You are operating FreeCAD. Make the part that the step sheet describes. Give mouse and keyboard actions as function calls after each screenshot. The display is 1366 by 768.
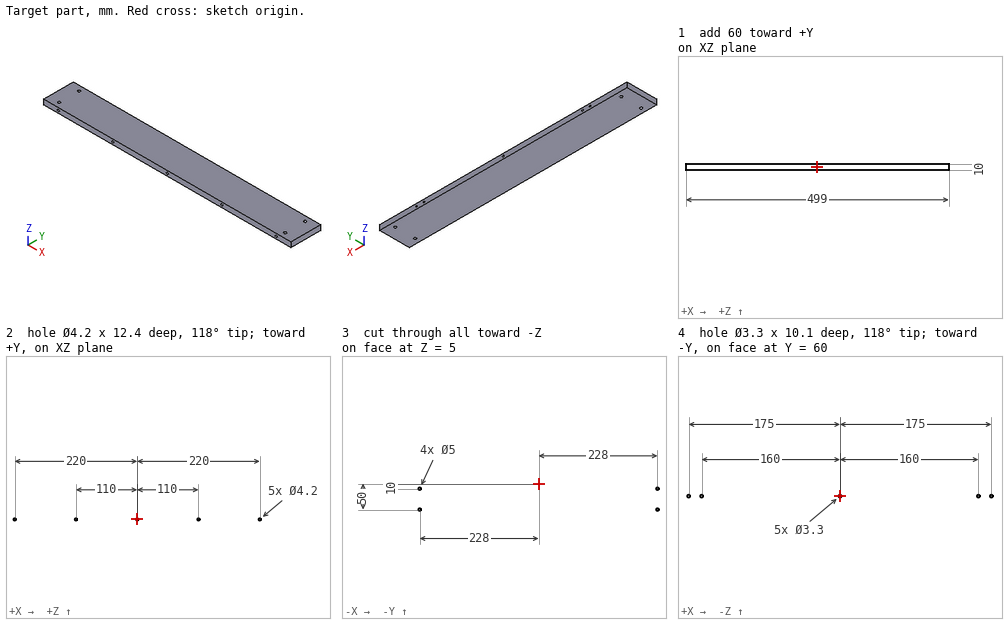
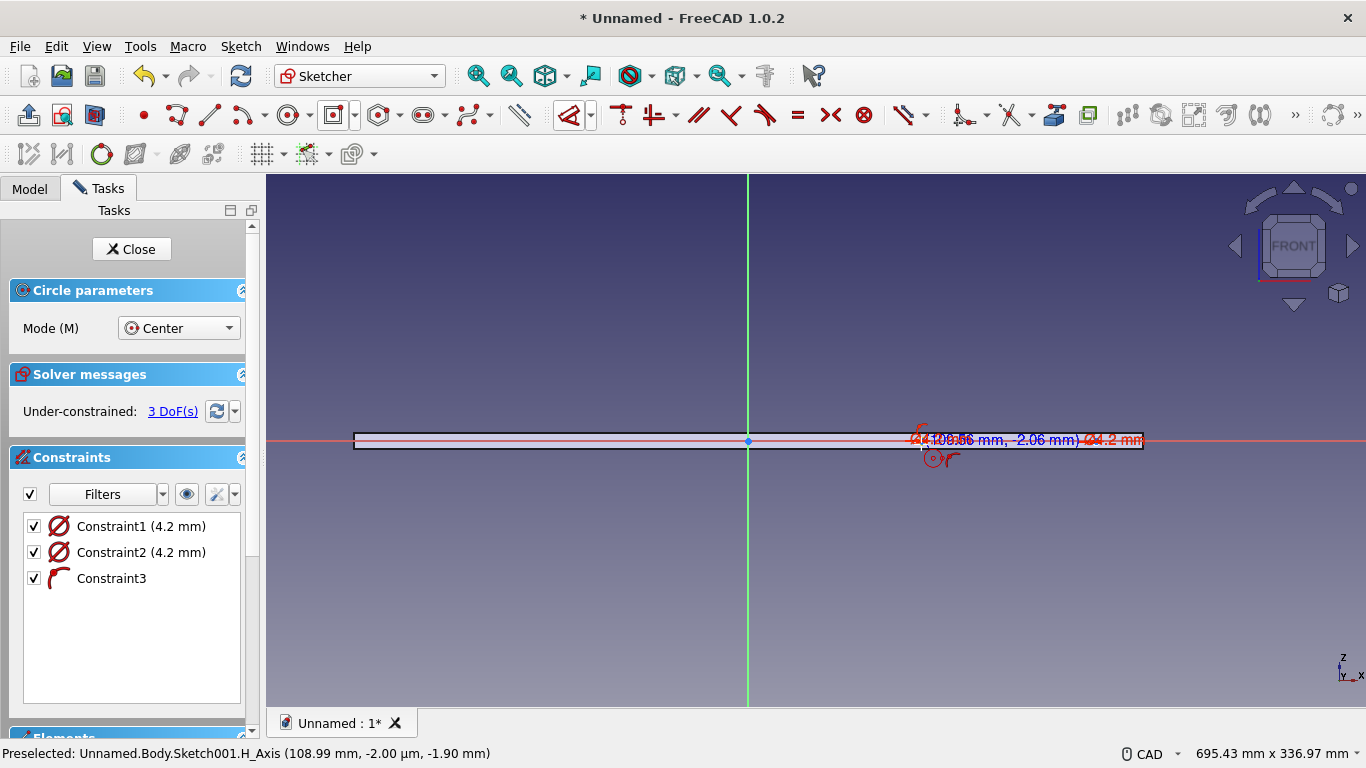
scroll(748, 441, up, 10)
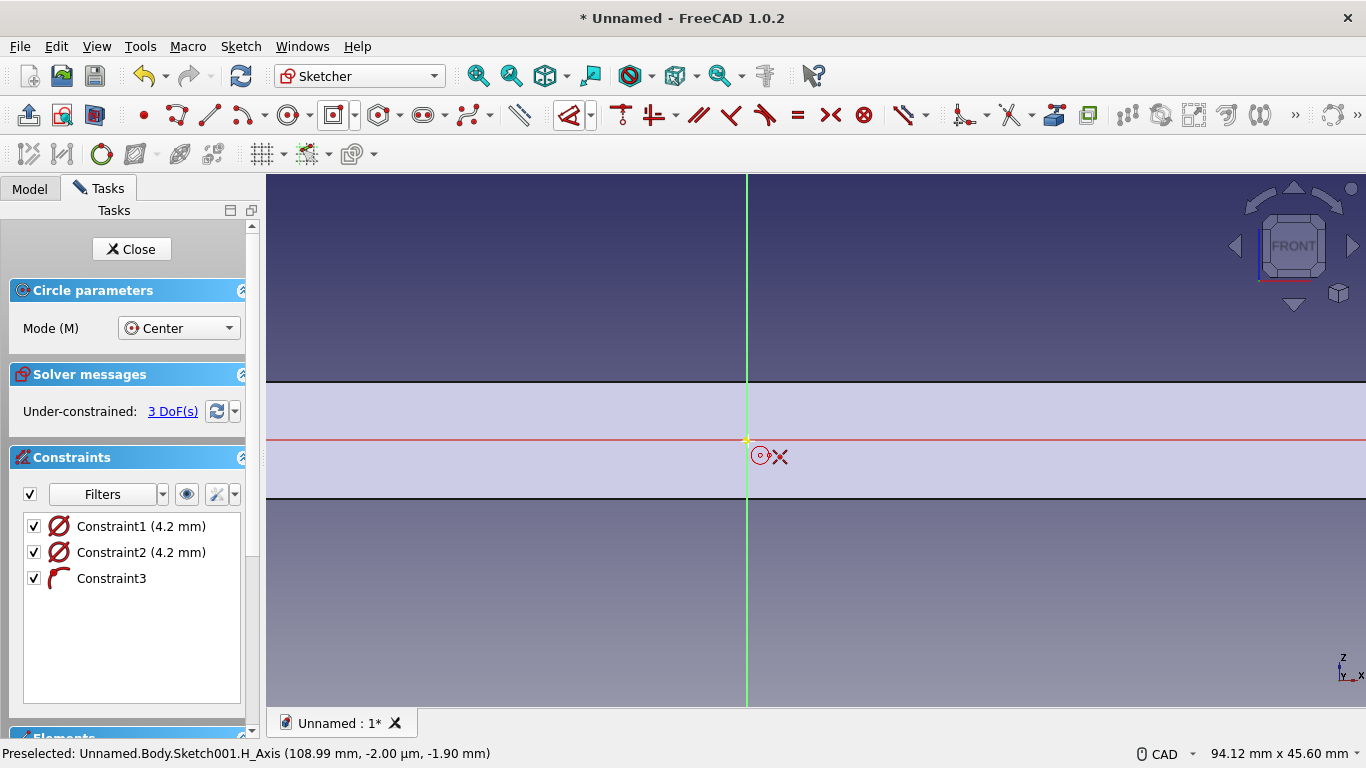
scroll(748, 441, down, 10)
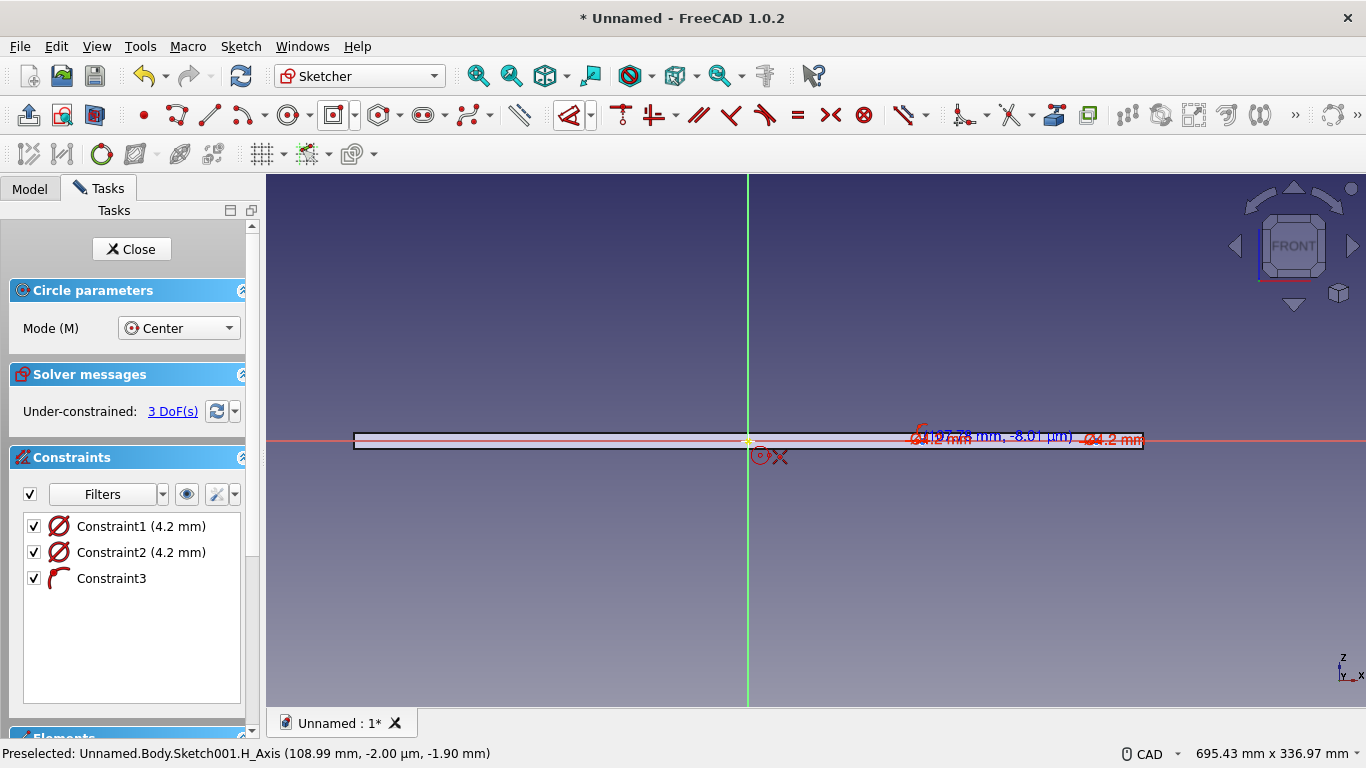
click(748, 441)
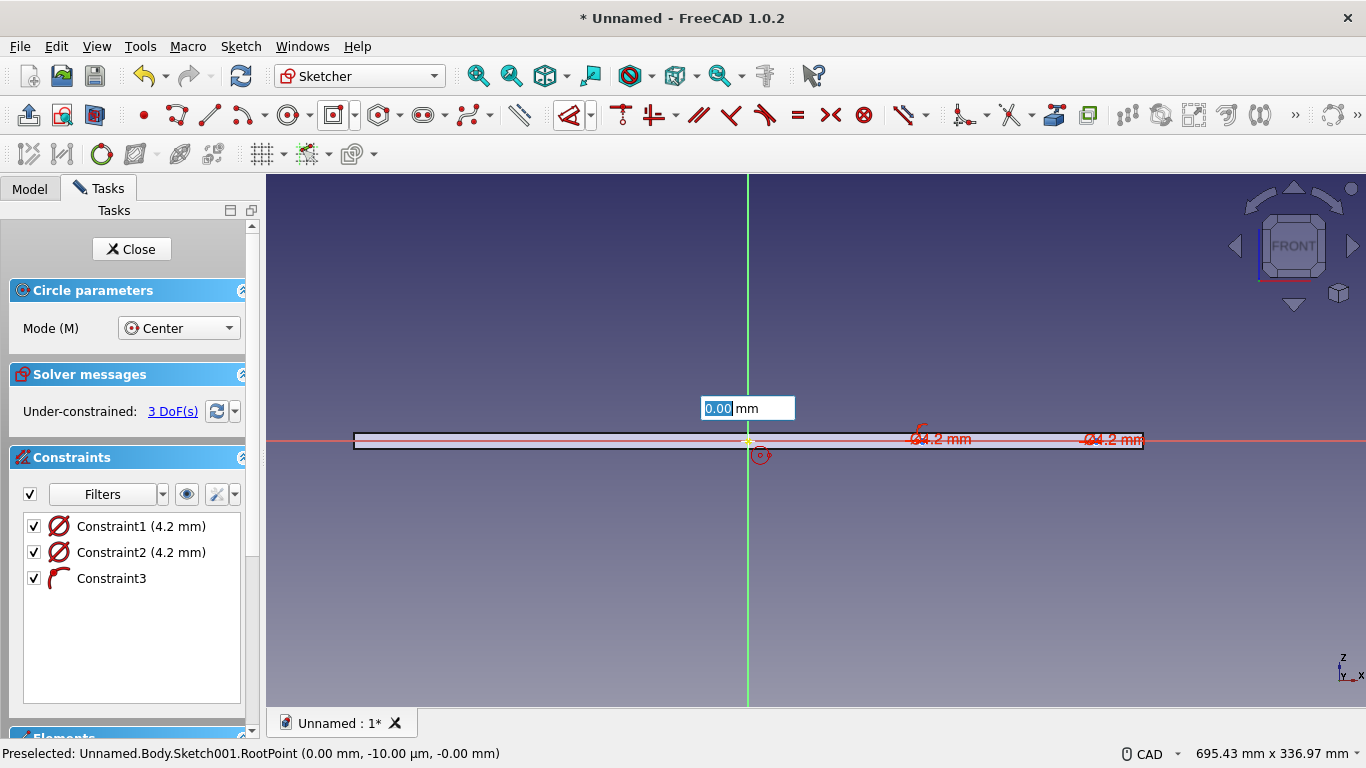
scroll(751, 439, up, 10)
move(745, 436)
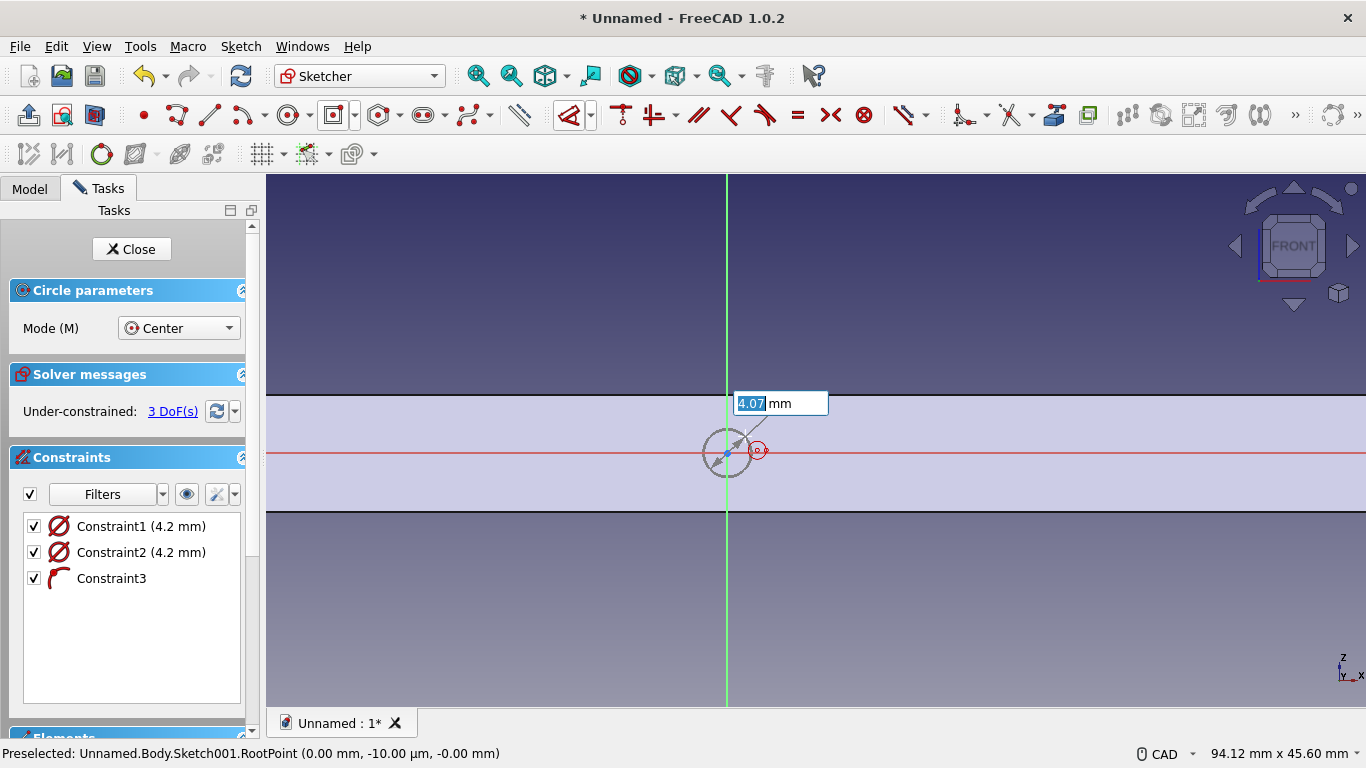
text(4.2)
key(Return)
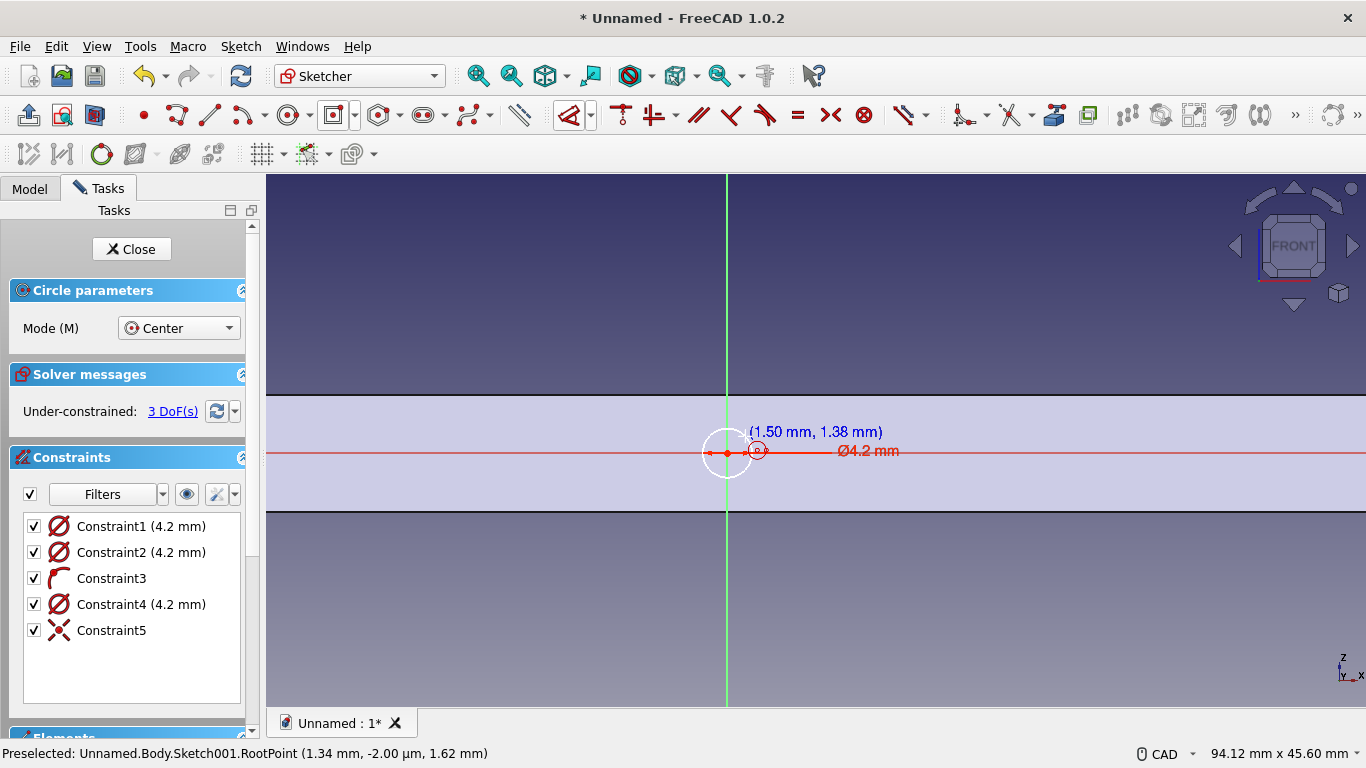
scroll(751, 439, down, 10)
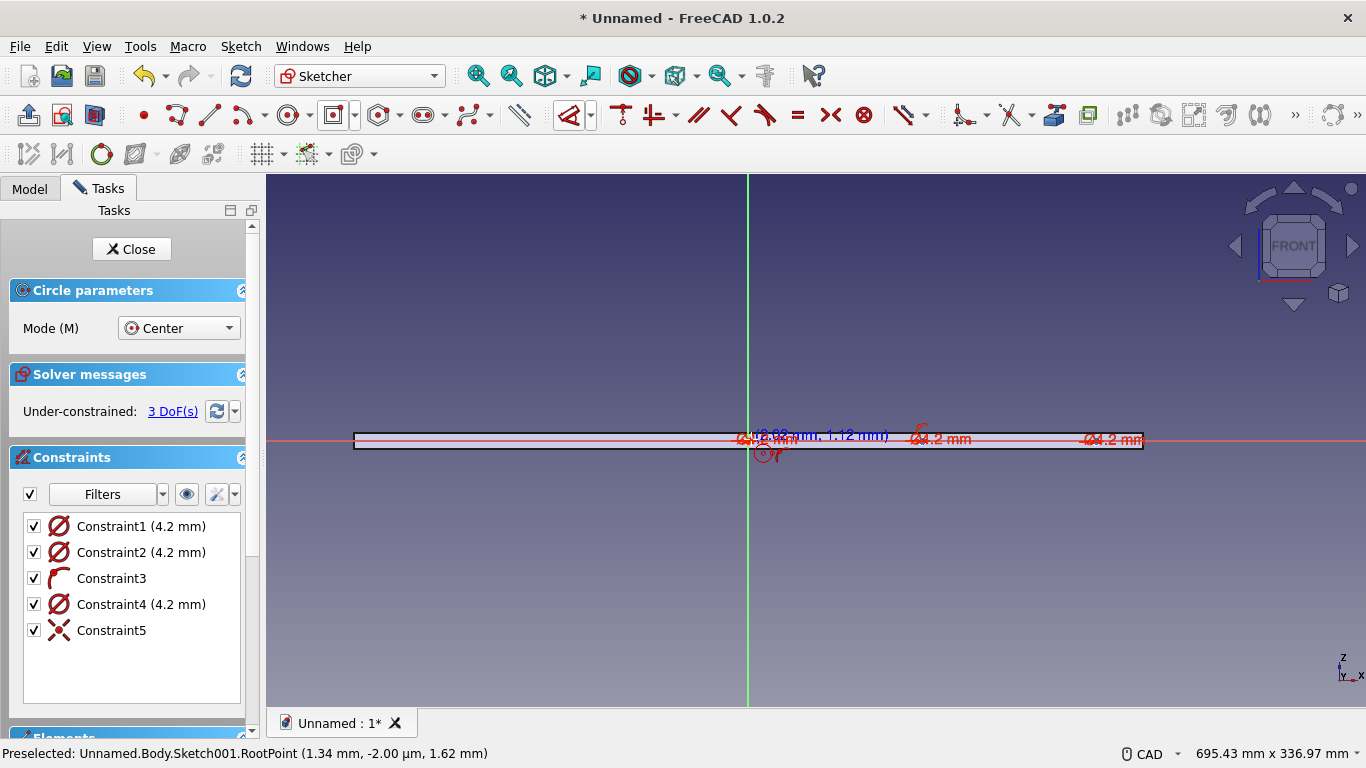
scroll(574, 441, up, 10)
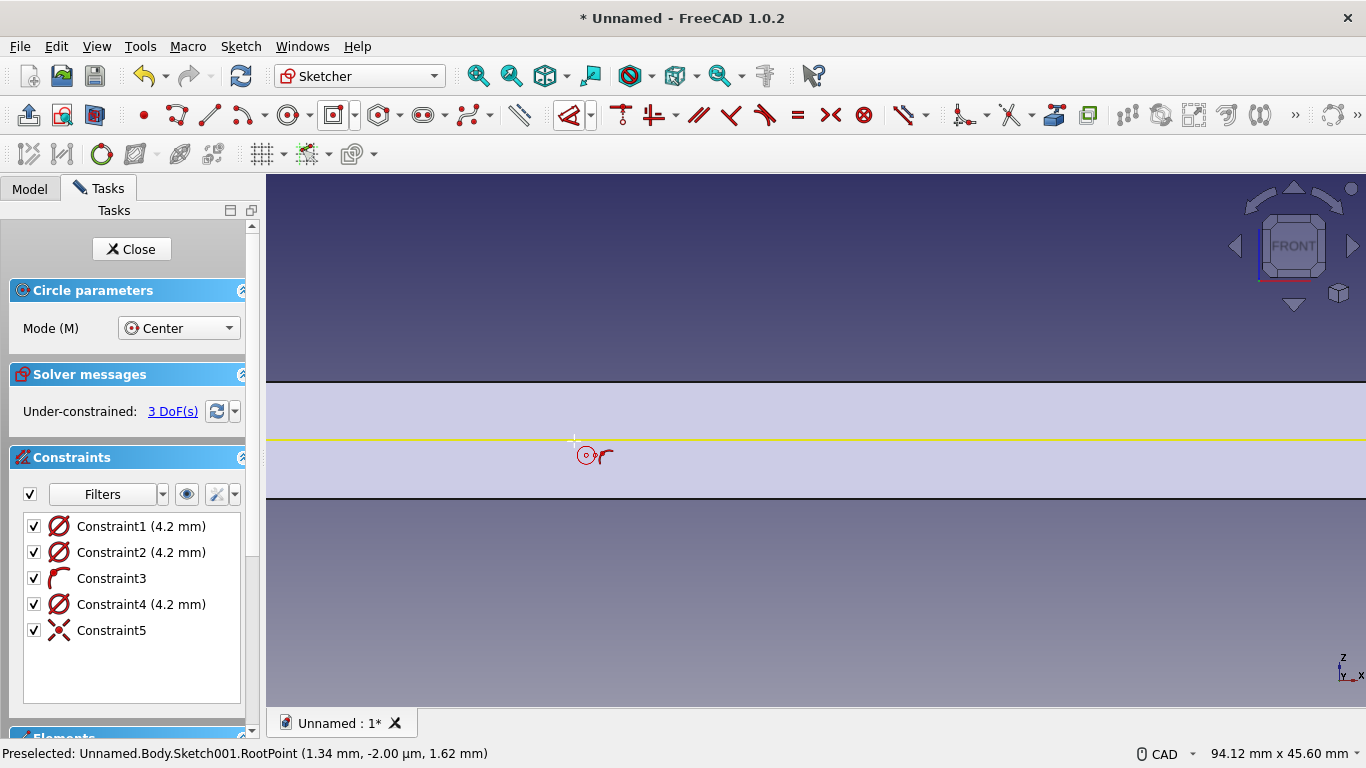
scroll(573, 441, down, 10)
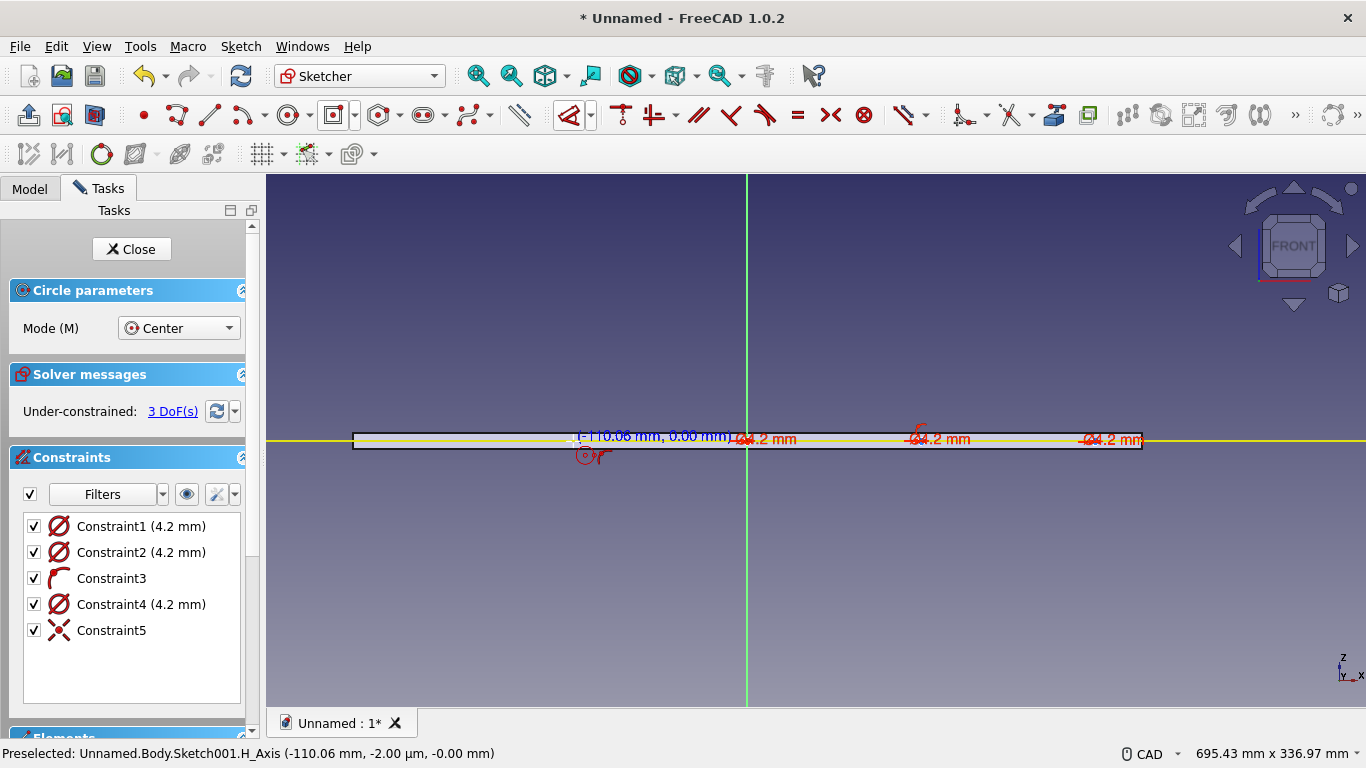
click(573, 441)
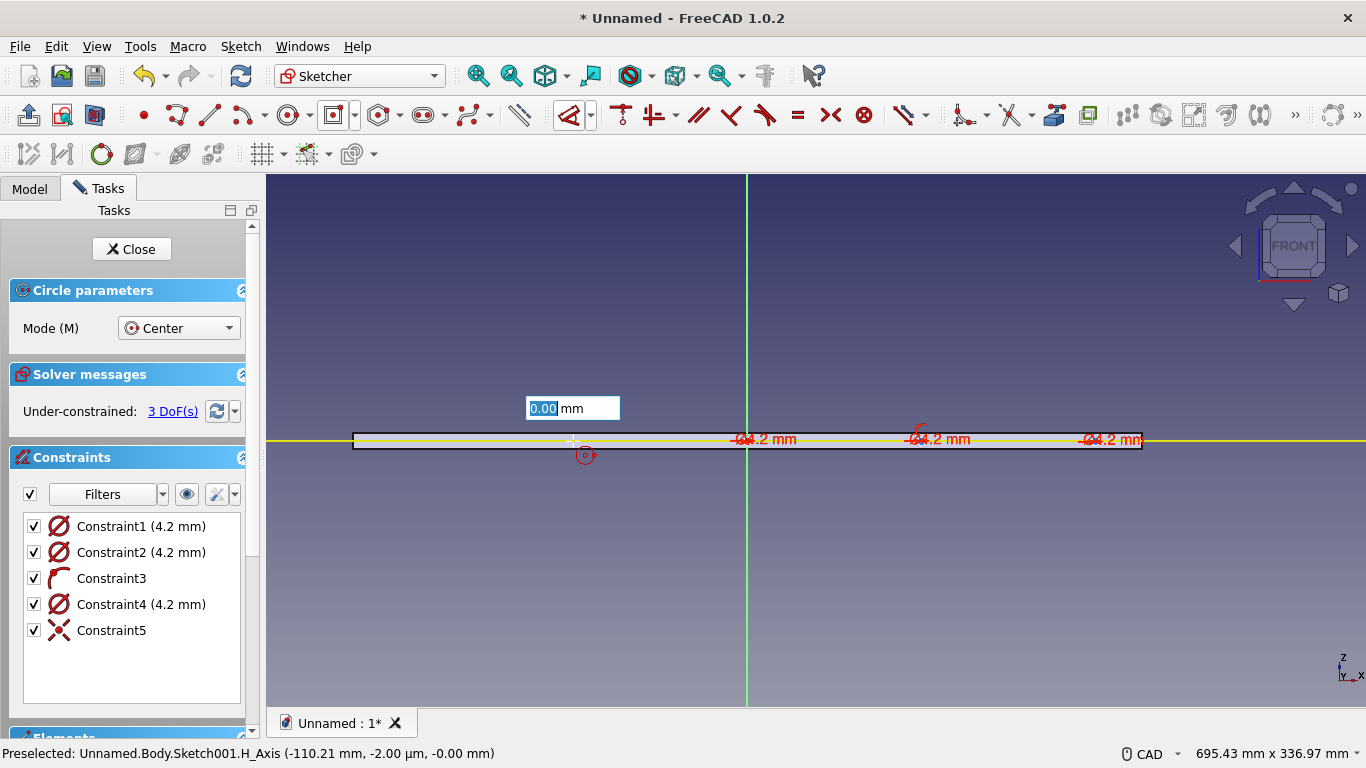
scroll(572, 444, up, 9)
move(572, 444)